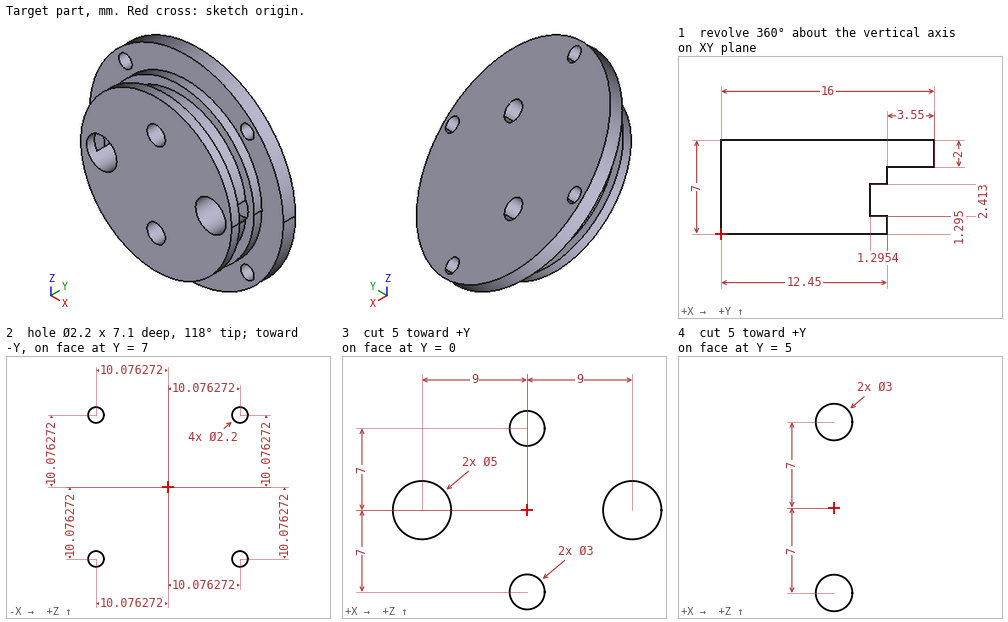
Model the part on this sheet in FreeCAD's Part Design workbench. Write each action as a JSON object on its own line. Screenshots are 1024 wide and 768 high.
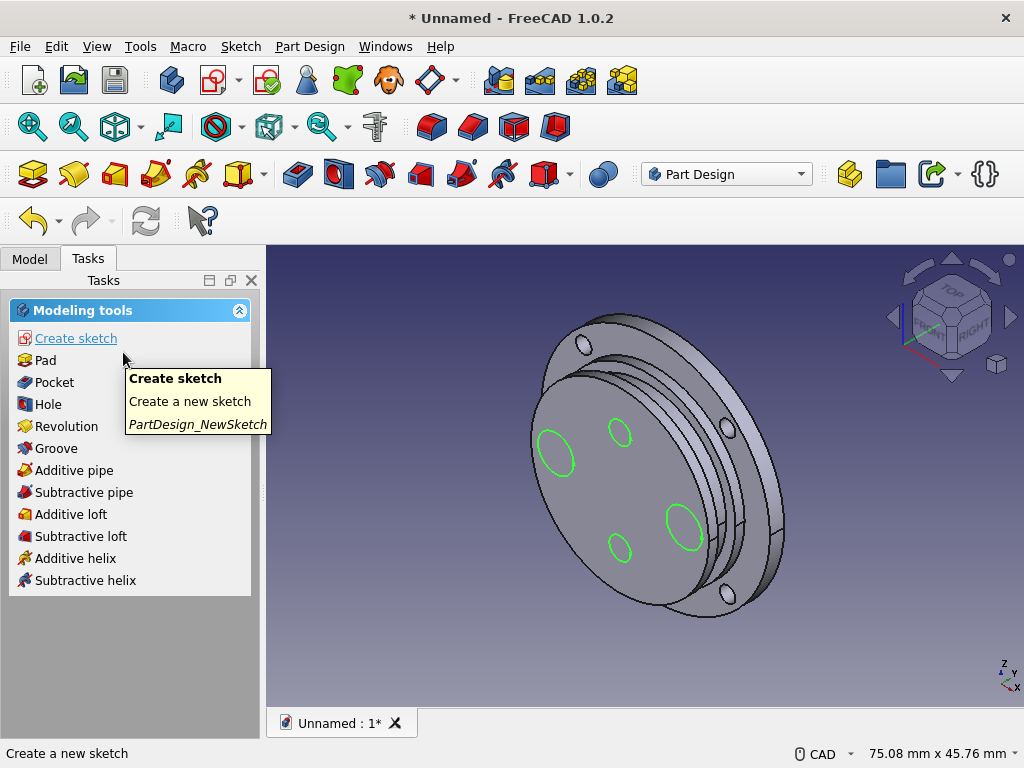
{"action": "left_click", "coordinate": [298, 174]}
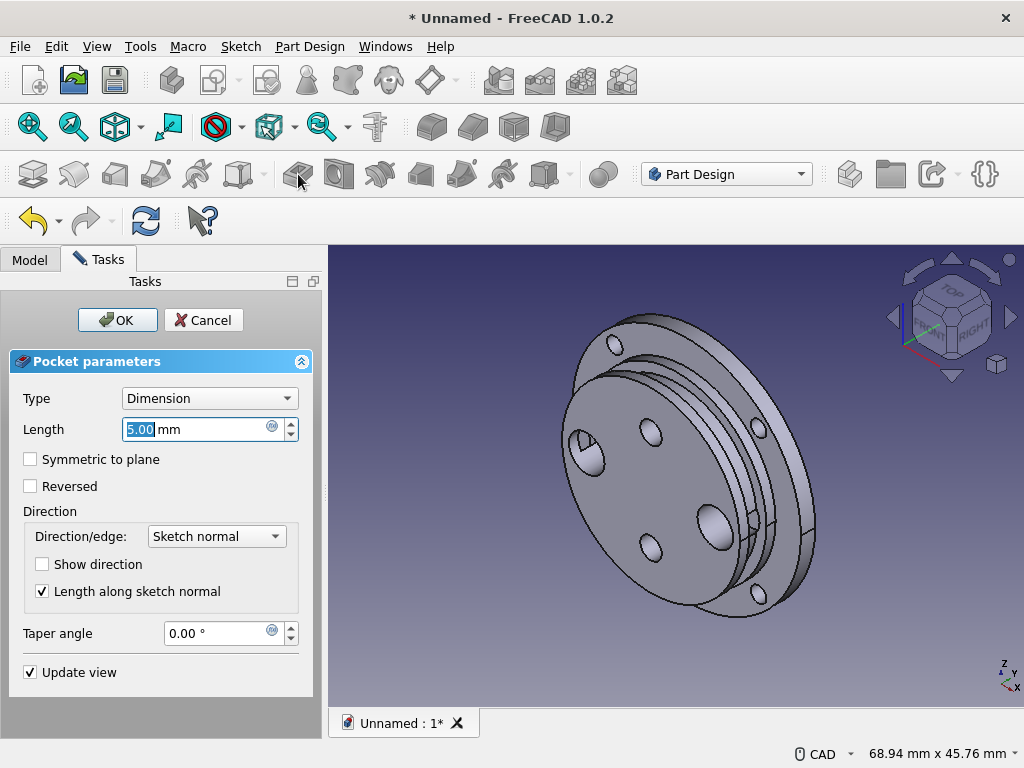
{"action": "type", "text": "5"}
{"action": "key", "text": "Tab"}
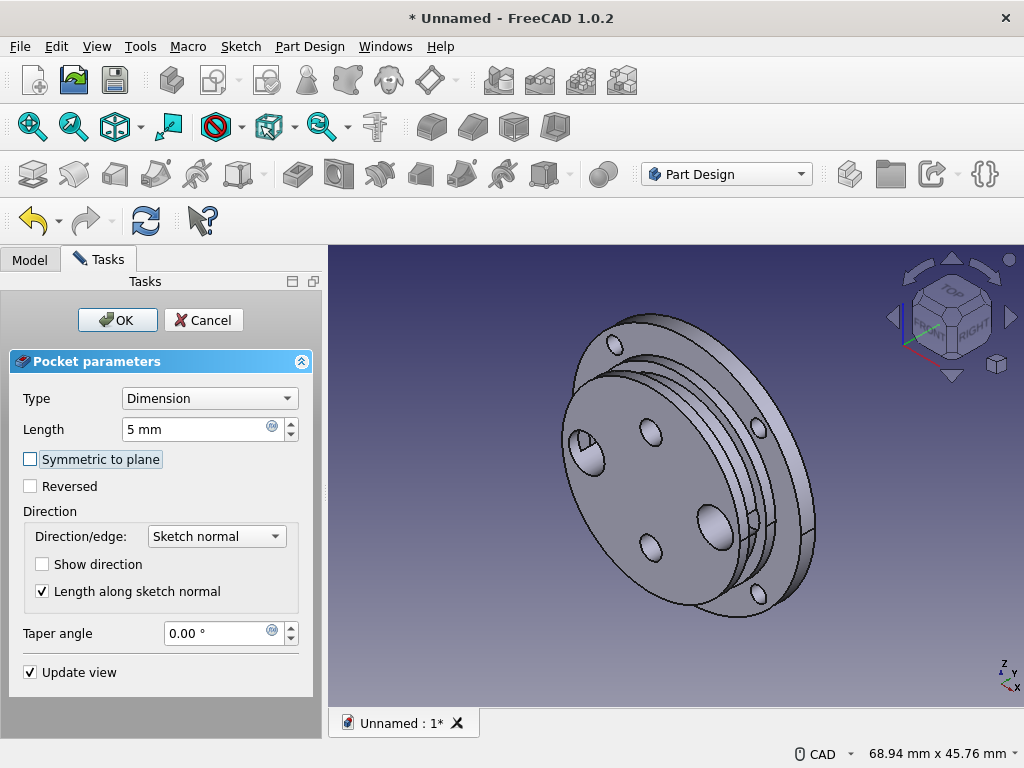
{"action": "left_click", "coordinate": [118, 320]}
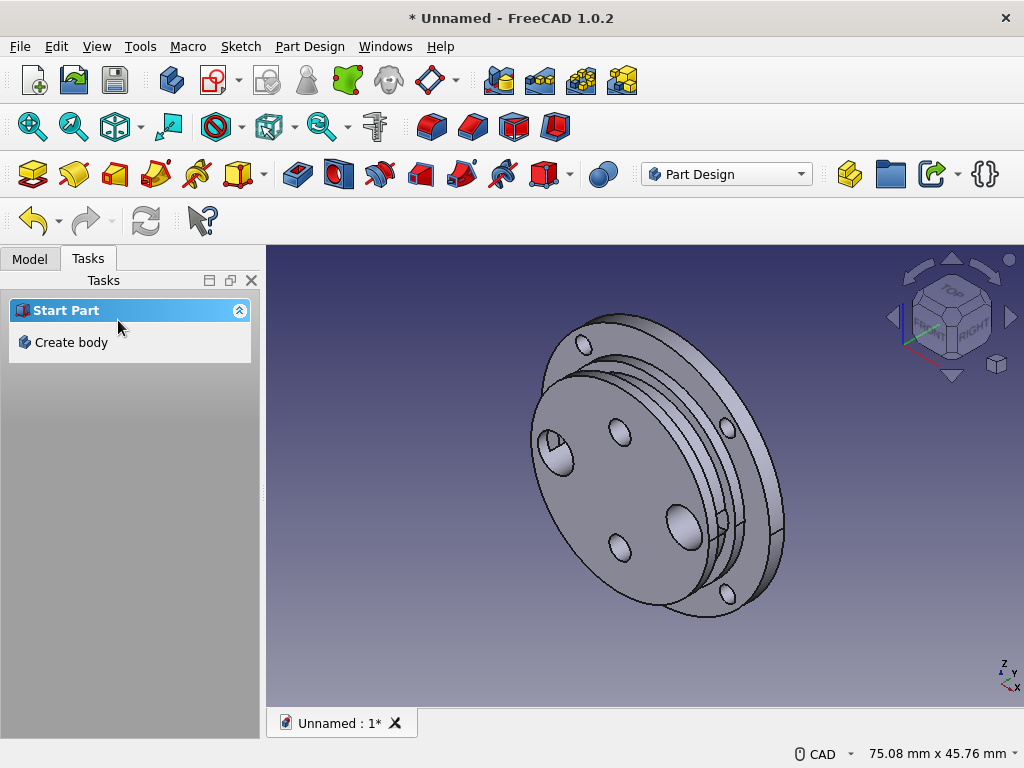
{"action": "left_click", "coordinate": [754, 563]}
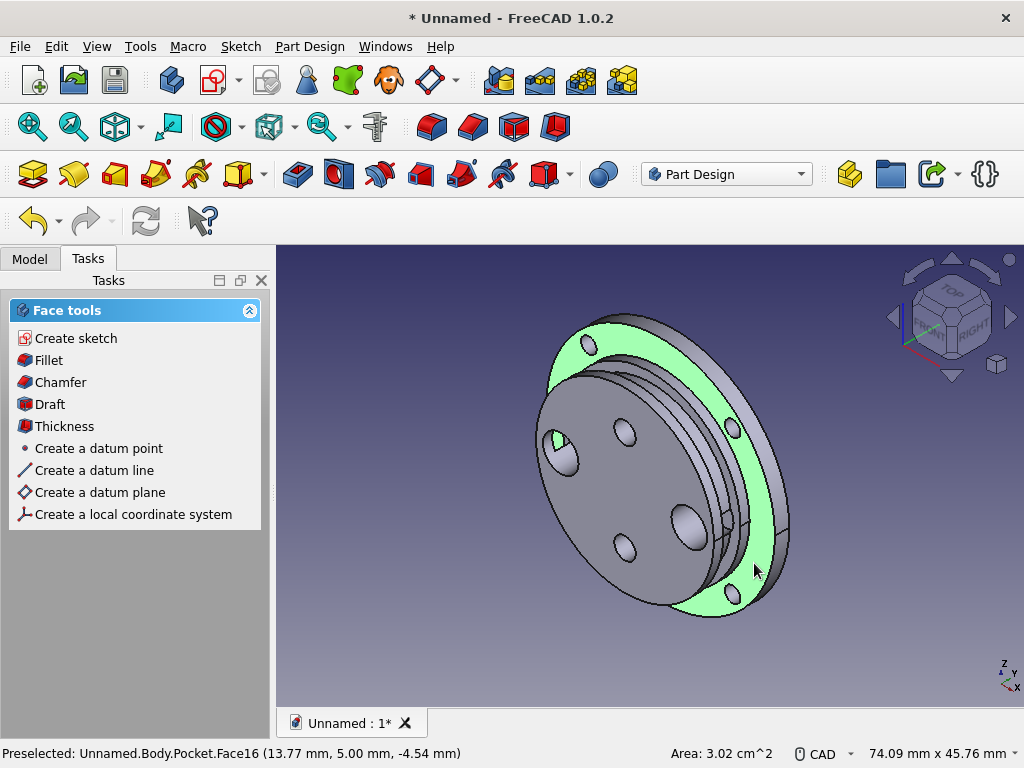
{"action": "left_click", "coordinate": [212, 80]}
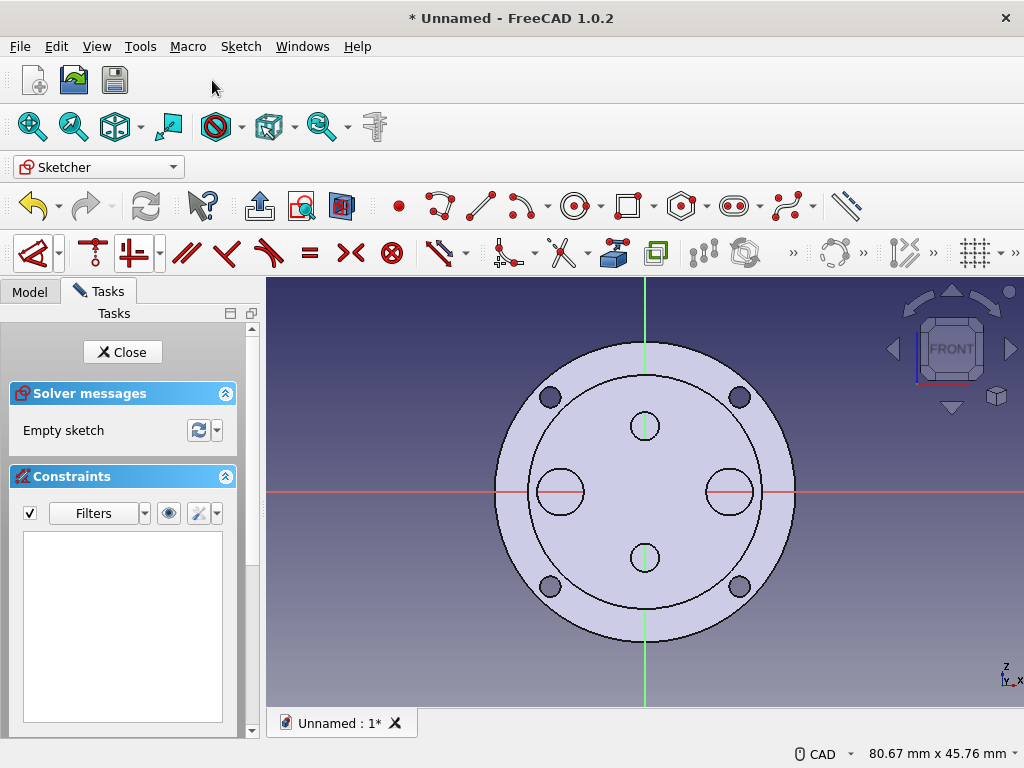
{"action": "scroll", "coordinate": [728, 492], "scroll_direction": "up", "scroll_amount": 3}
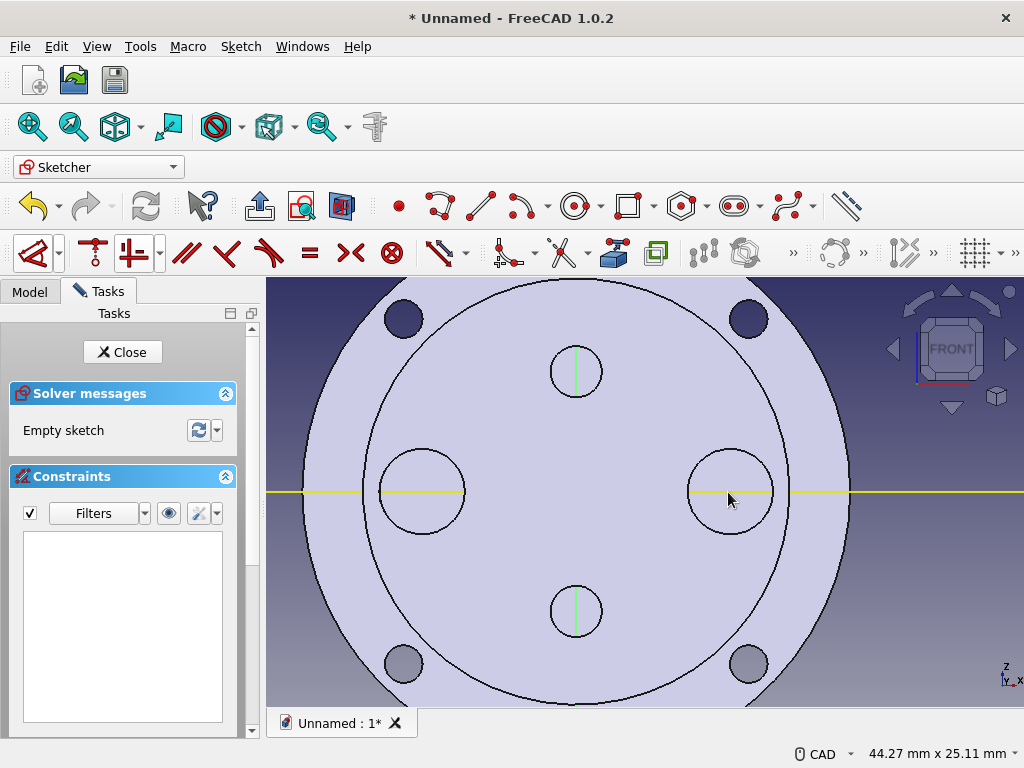
{"action": "left_click", "coordinate": [574, 206]}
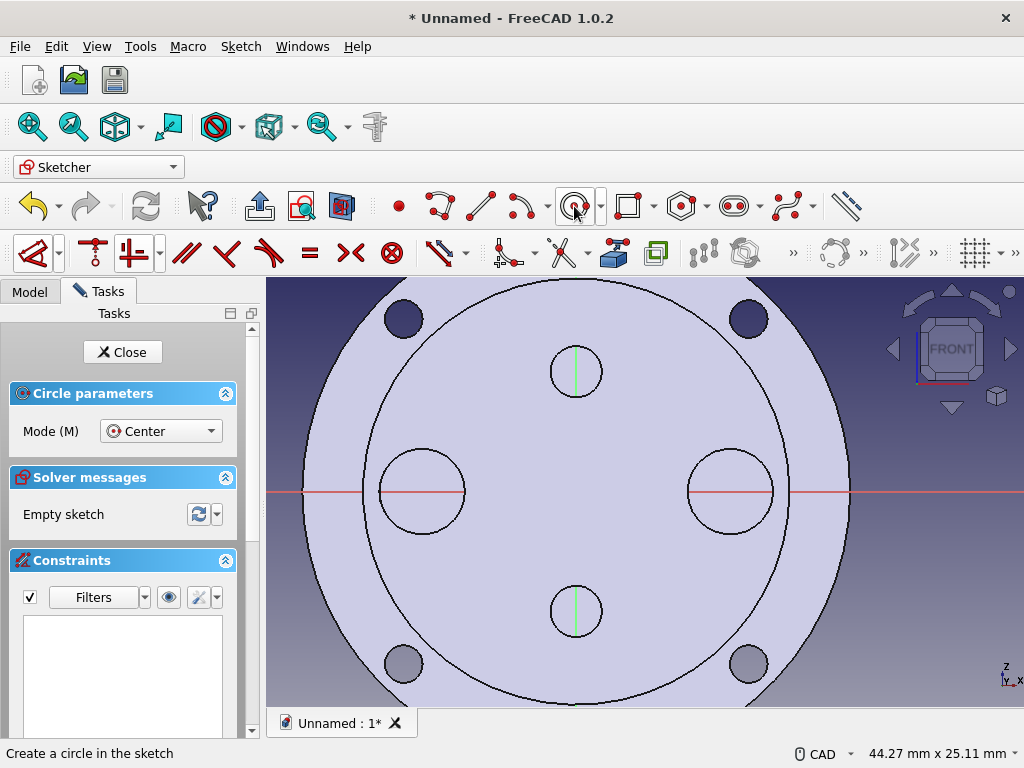
{"action": "left_click", "coordinate": [576, 372]}
{"action": "mouse_move", "coordinate": [594, 354]}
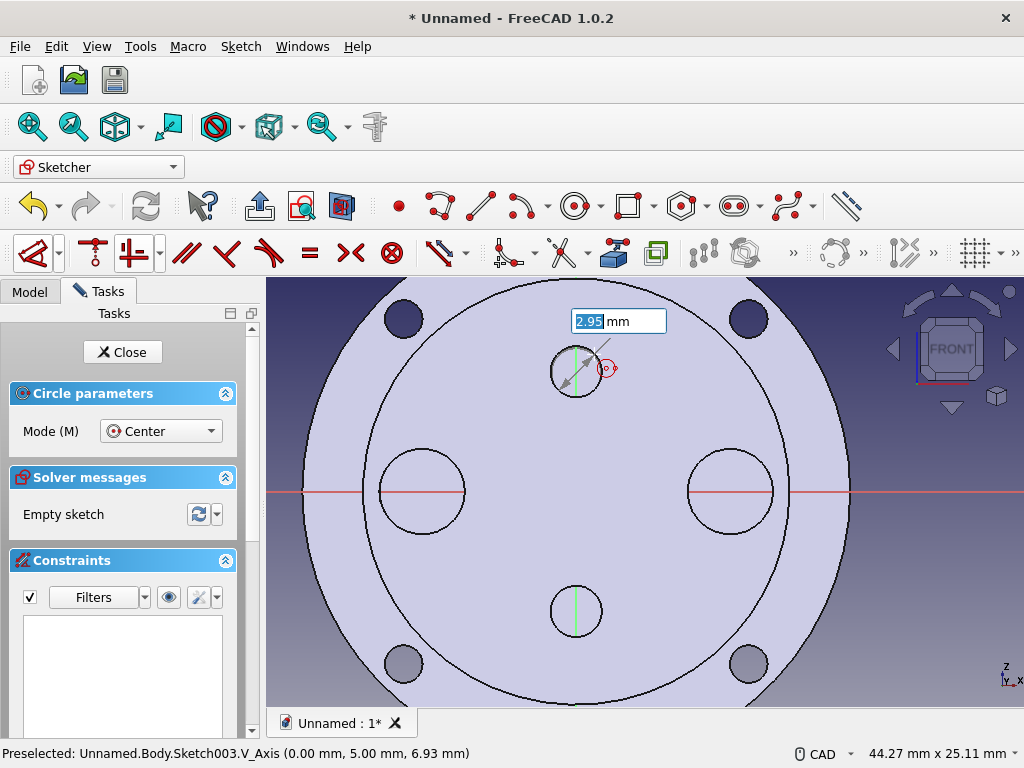
{"action": "type", "text": "3"}
{"action": "key", "text": "Return"}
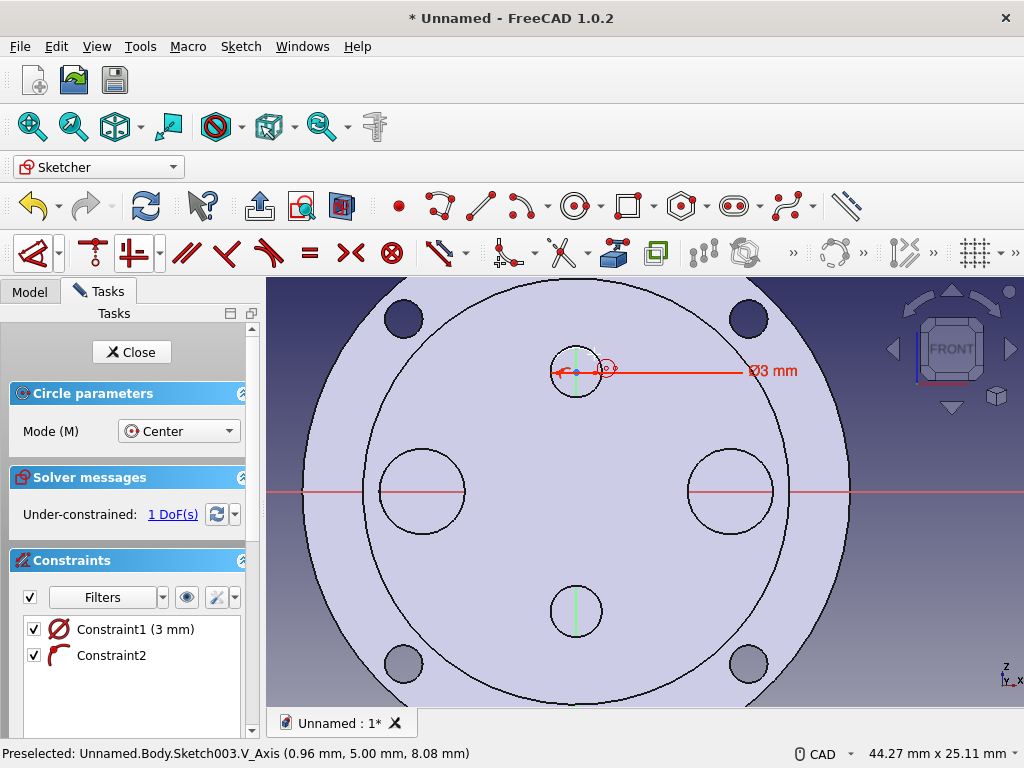
{"action": "left_click", "coordinate": [576, 611]}
{"action": "mouse_move", "coordinate": [594, 593]}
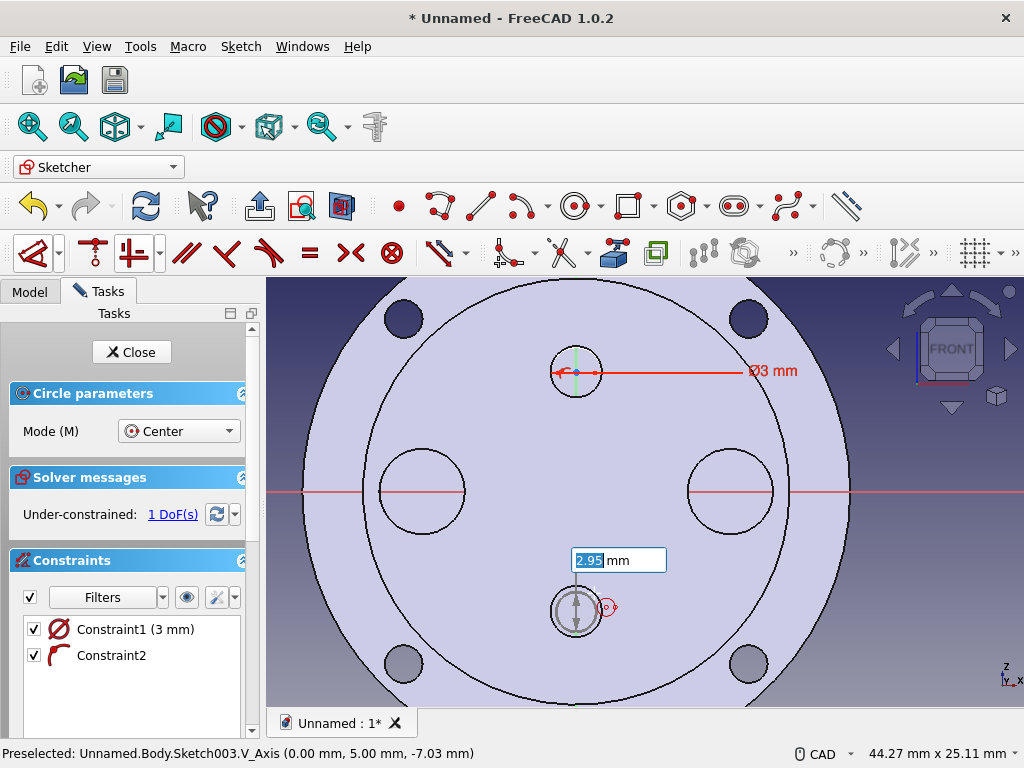
{"action": "type", "text": "3"}
{"action": "key", "text": "Return"}
{"action": "key", "text": "Escape"}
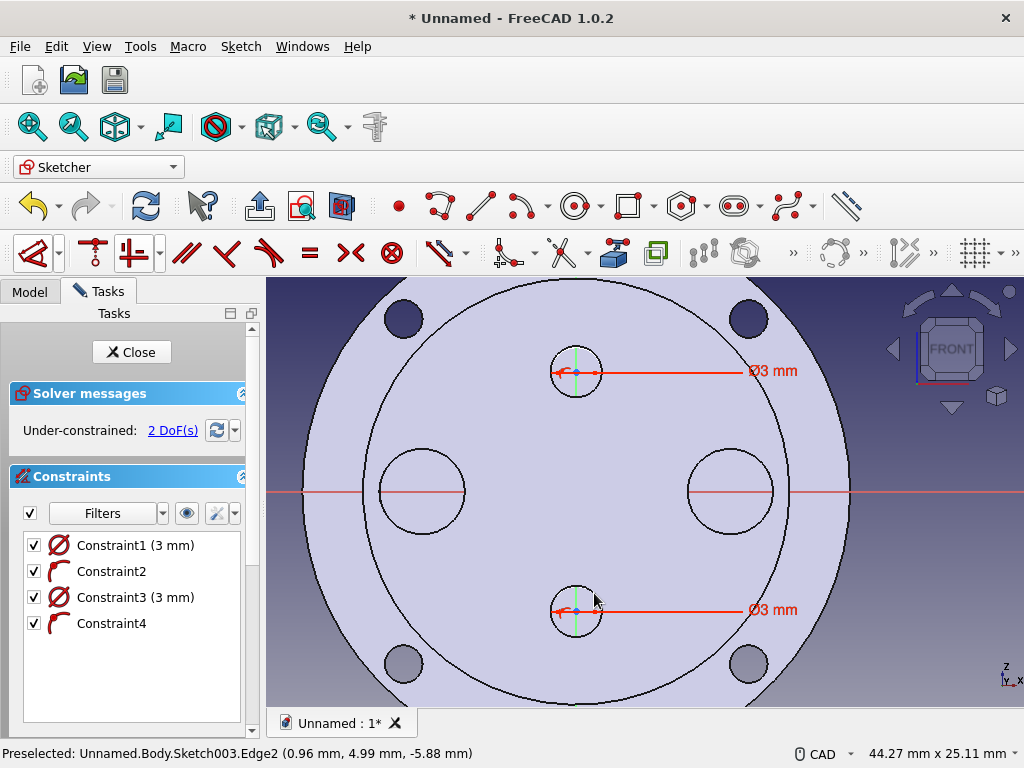
{"action": "left_click", "coordinate": [576, 373]}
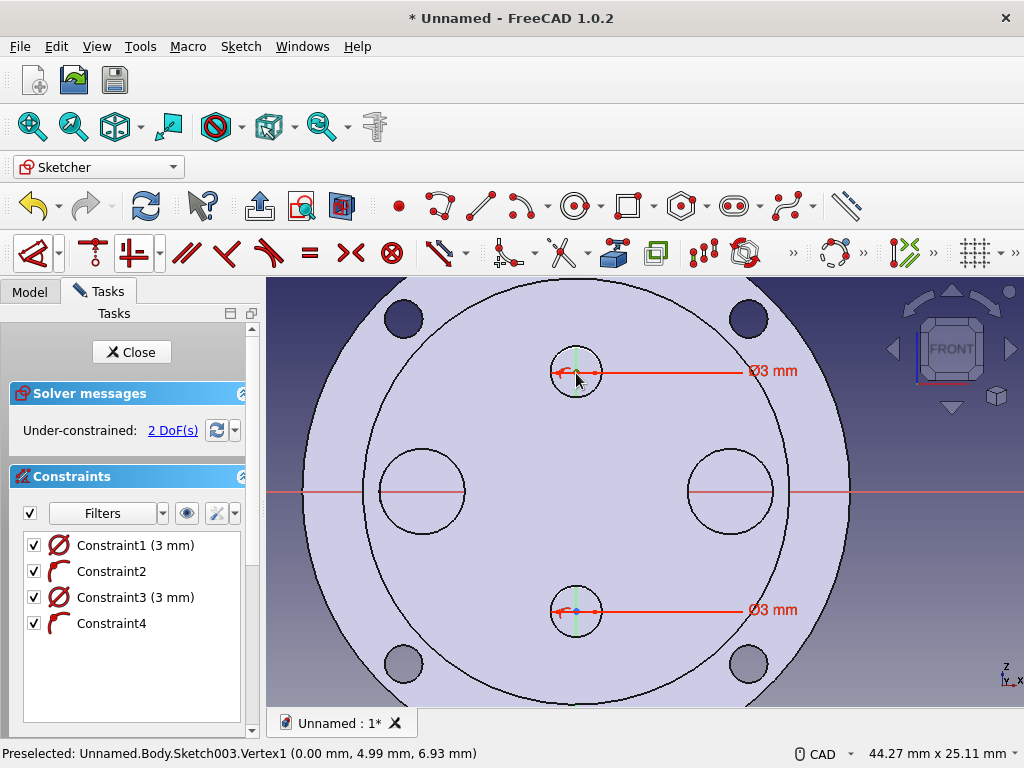
{"action": "left_click", "coordinate": [58, 254]}